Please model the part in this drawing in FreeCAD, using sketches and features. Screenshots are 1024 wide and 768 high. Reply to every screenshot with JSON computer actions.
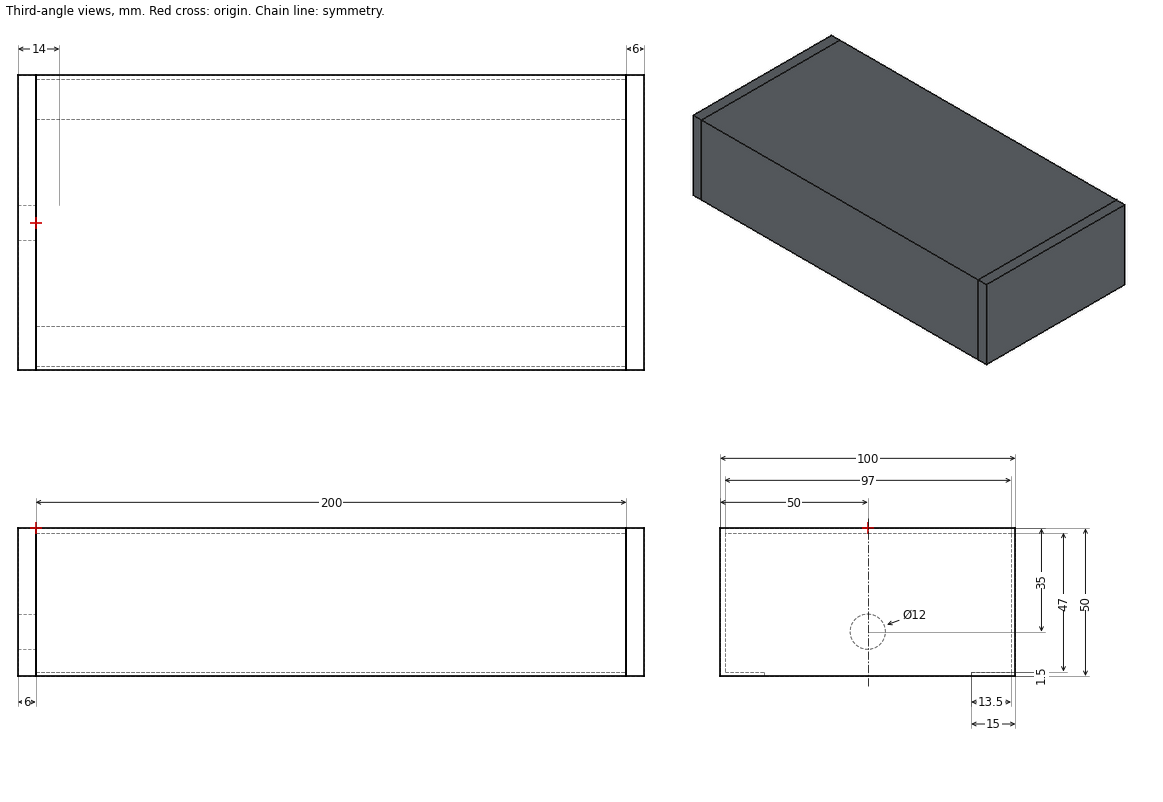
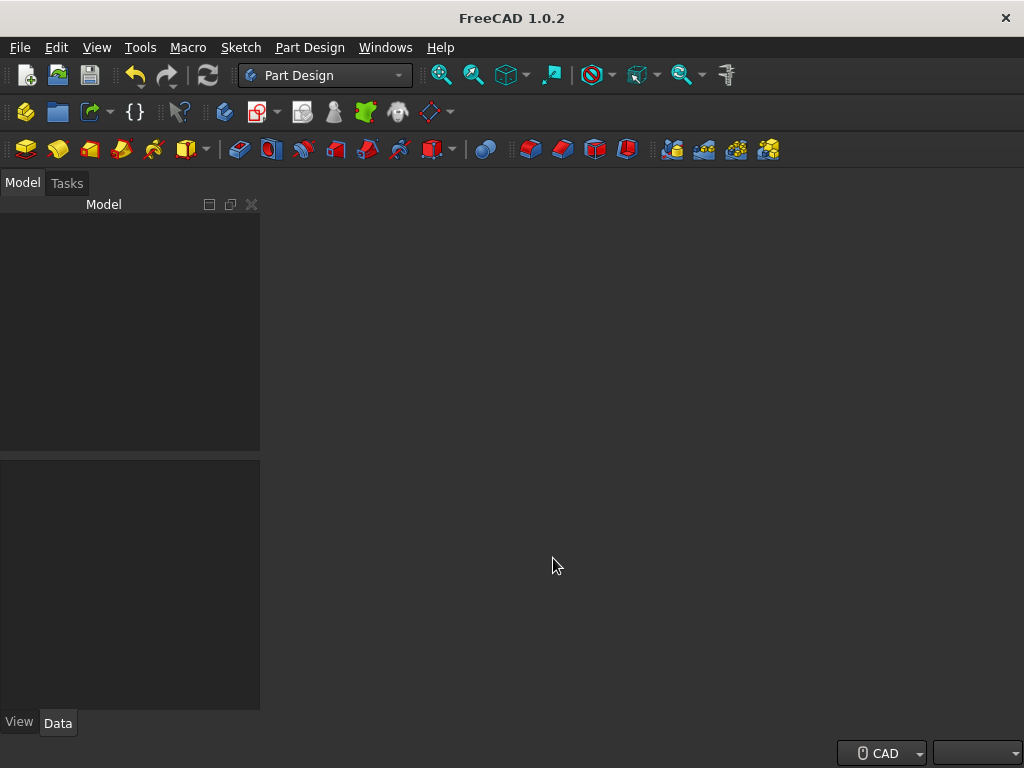
{"action": "left_click", "coordinate": [26, 76]}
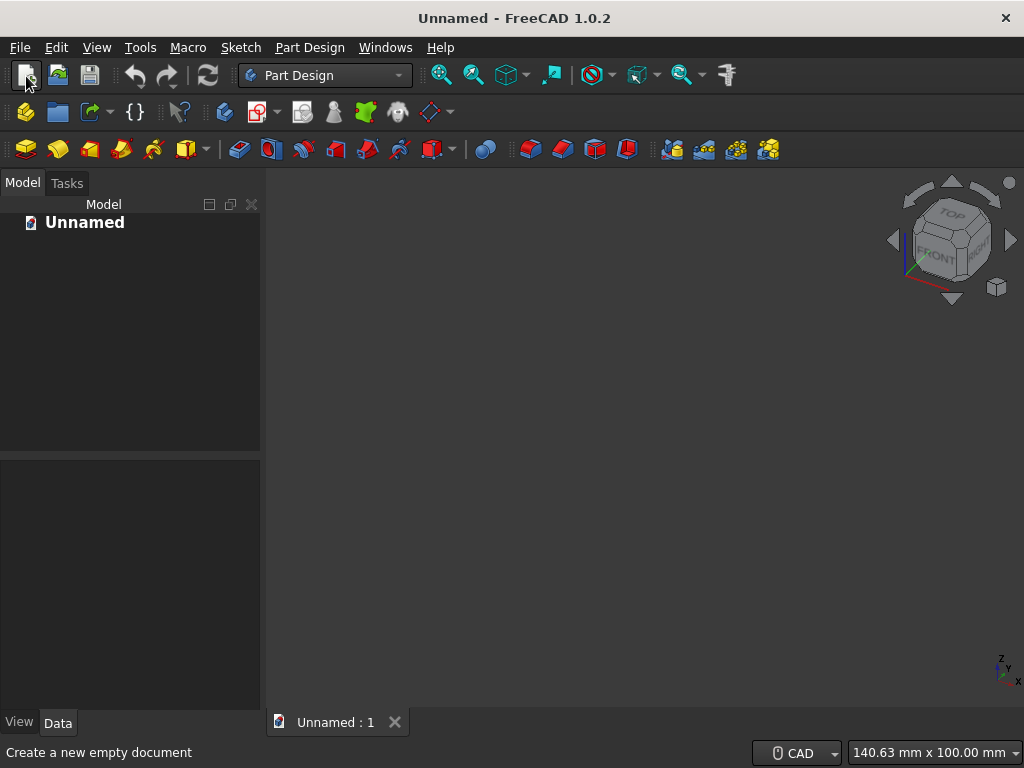
{"action": "left_click", "coordinate": [258, 112]}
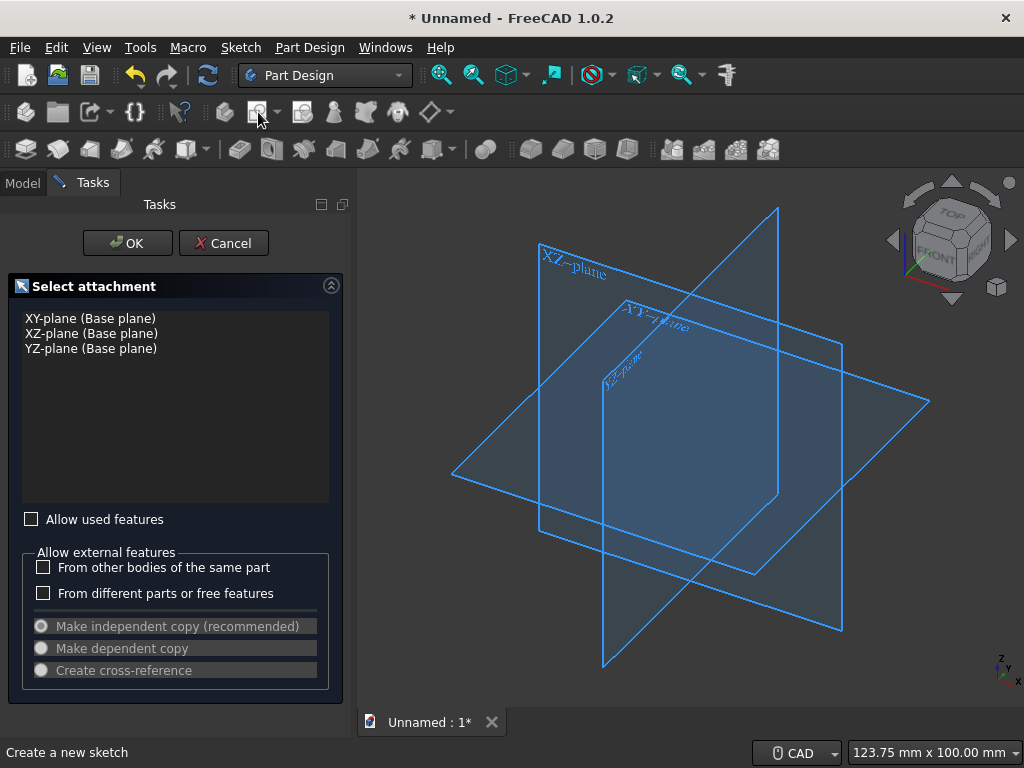
{"action": "left_click", "coordinate": [82, 348]}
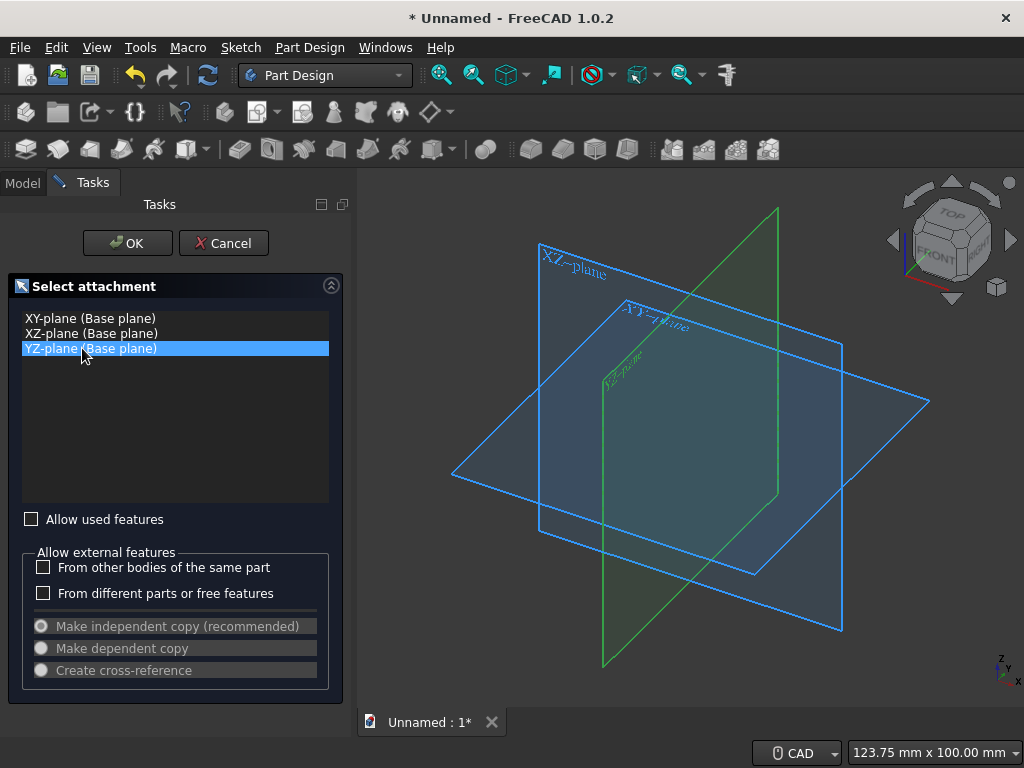
{"action": "left_click", "coordinate": [128, 243]}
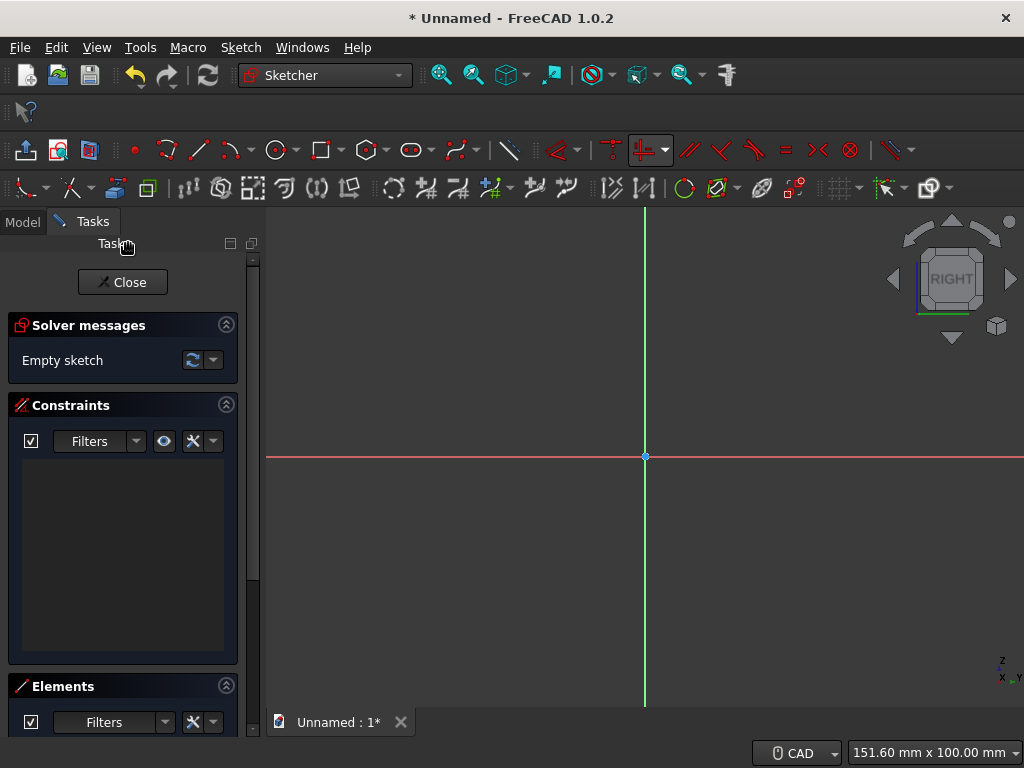
{"action": "scroll", "coordinate": [294, 235], "scroll_direction": "down", "scroll_amount": 1}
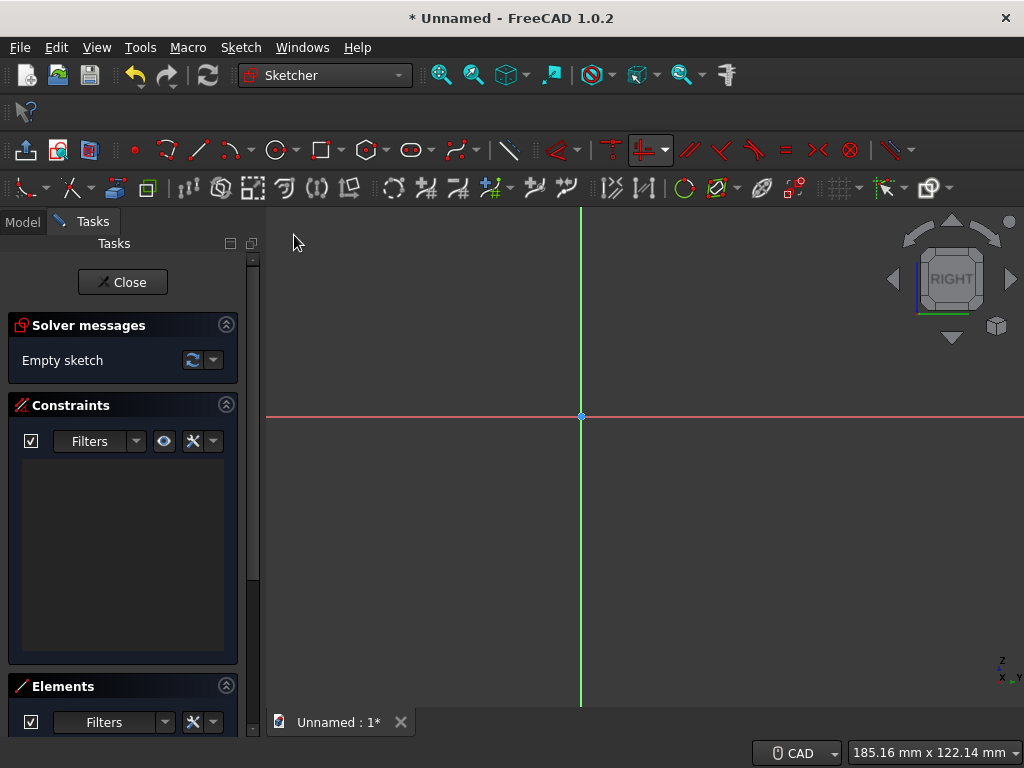
{"action": "left_click", "coordinate": [168, 150]}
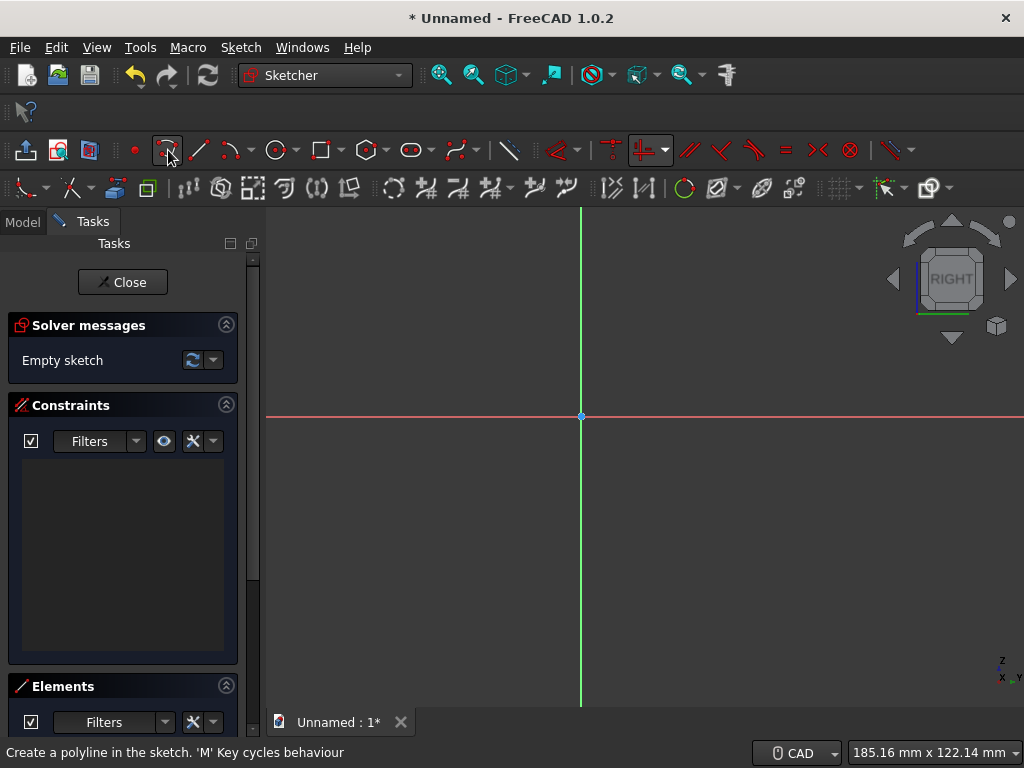
{"action": "scroll", "coordinate": [383, 423], "scroll_direction": "up", "scroll_amount": 5}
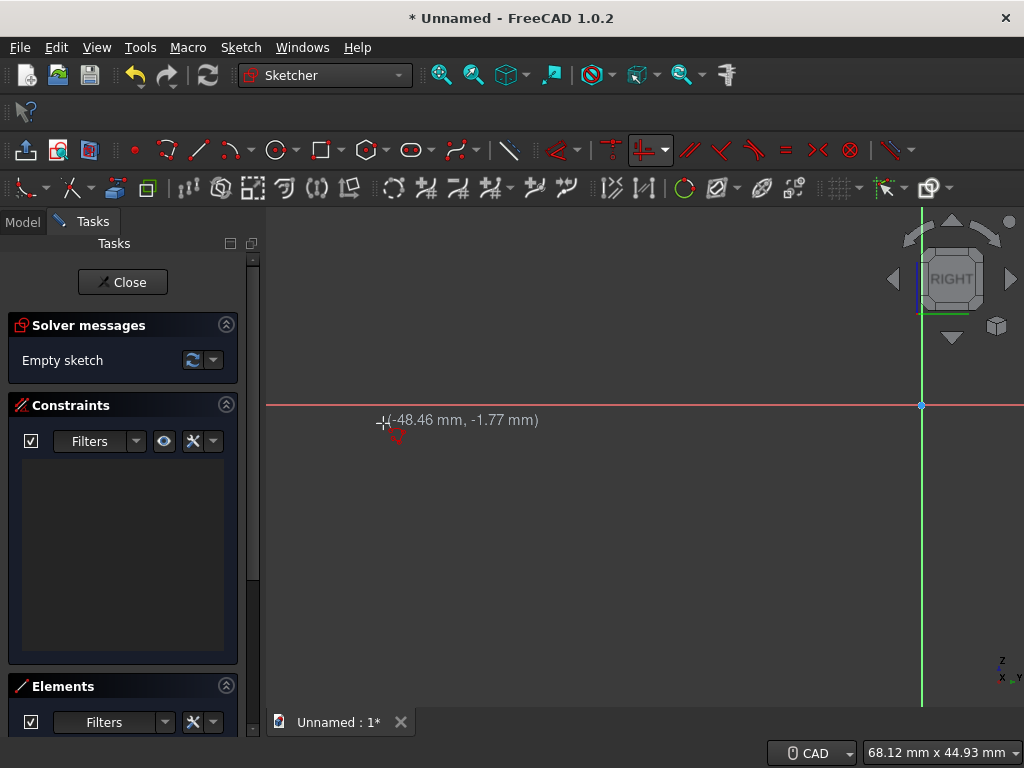
{"action": "left_click", "coordinate": [382, 422]}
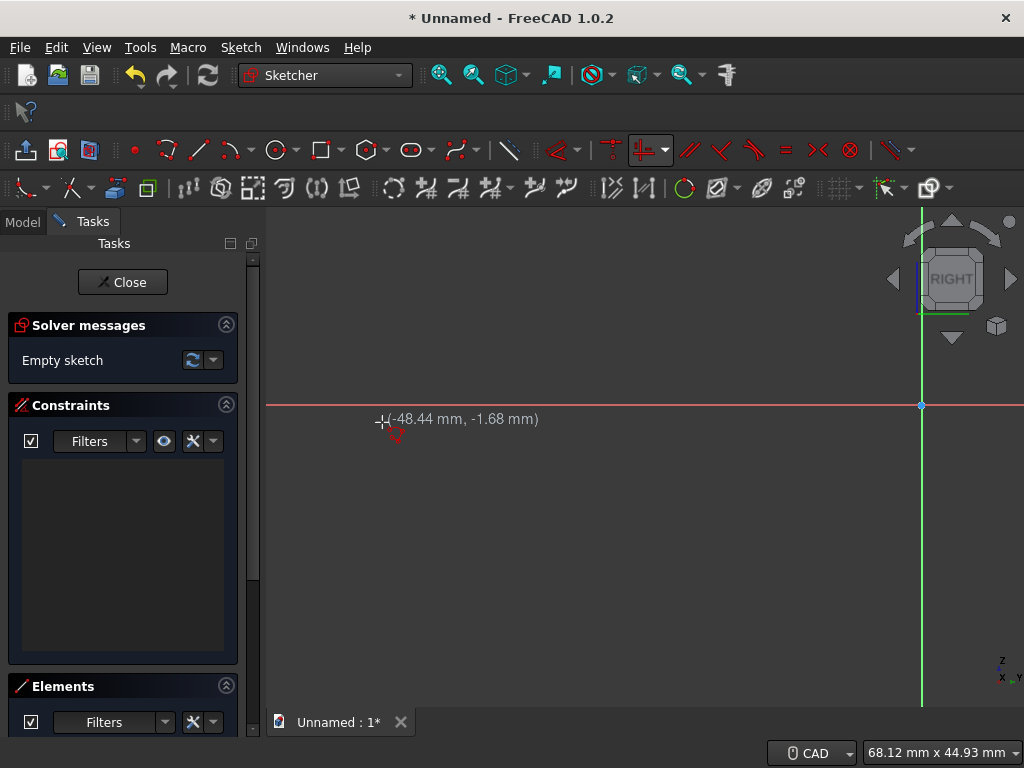
{"action": "scroll", "coordinate": [375, 325], "scroll_direction": "down", "scroll_amount": 5}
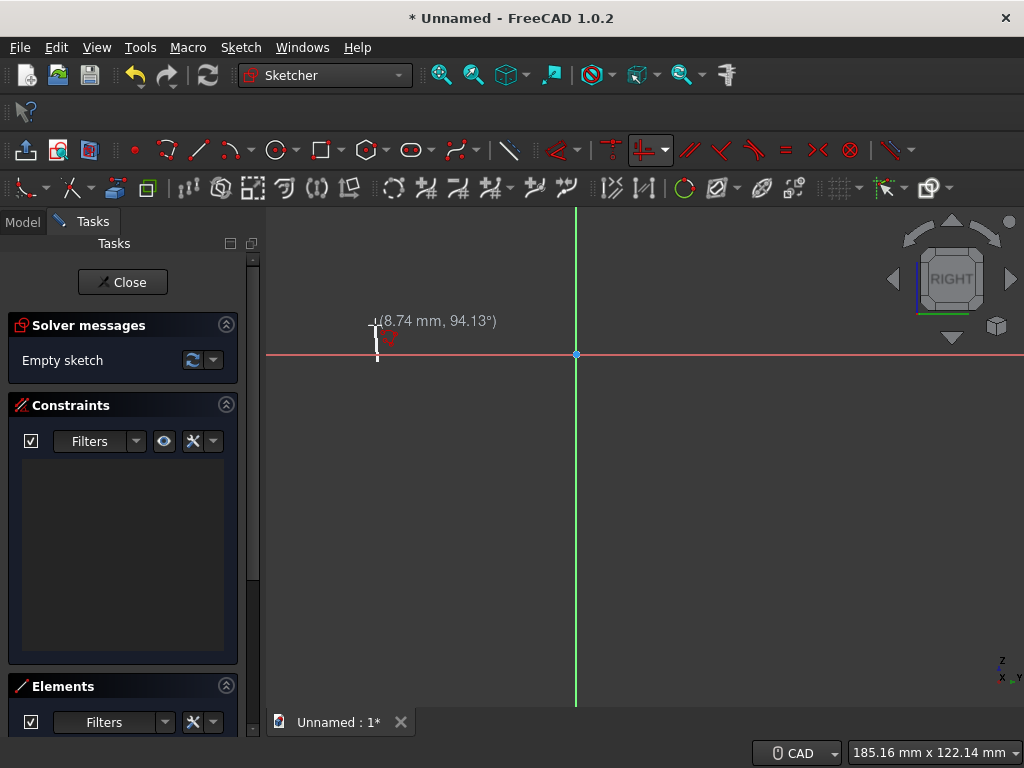
{"action": "scroll", "coordinate": [775, 361], "scroll_direction": "up", "scroll_amount": 5}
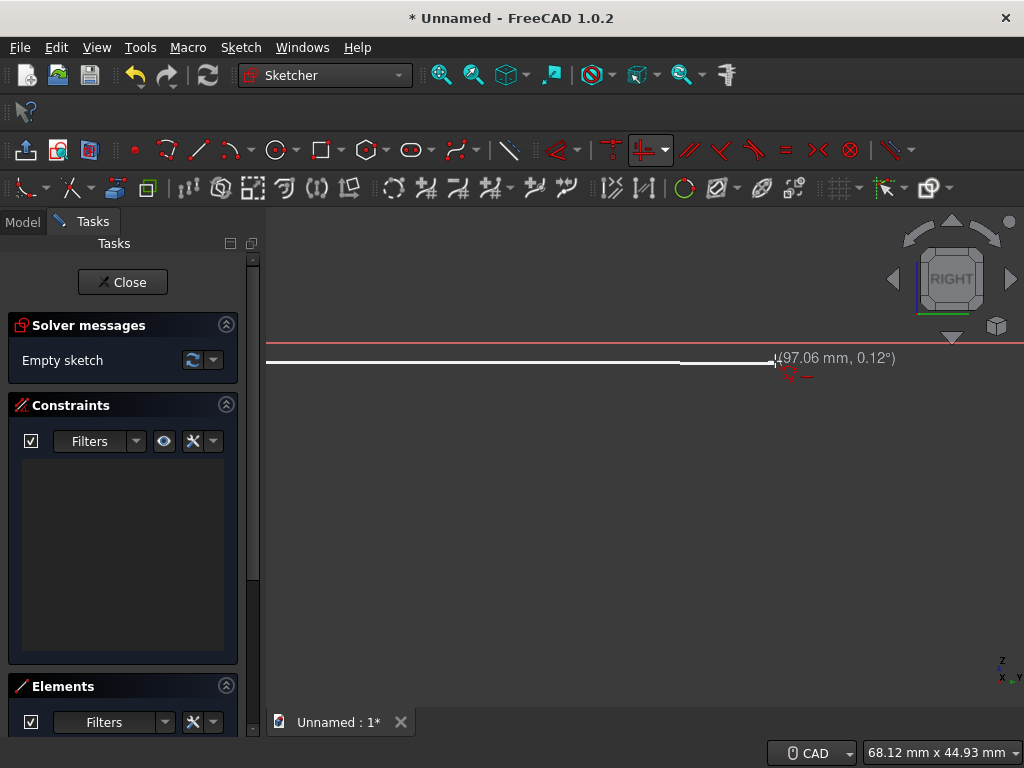
{"action": "left_click", "coordinate": [773, 360]}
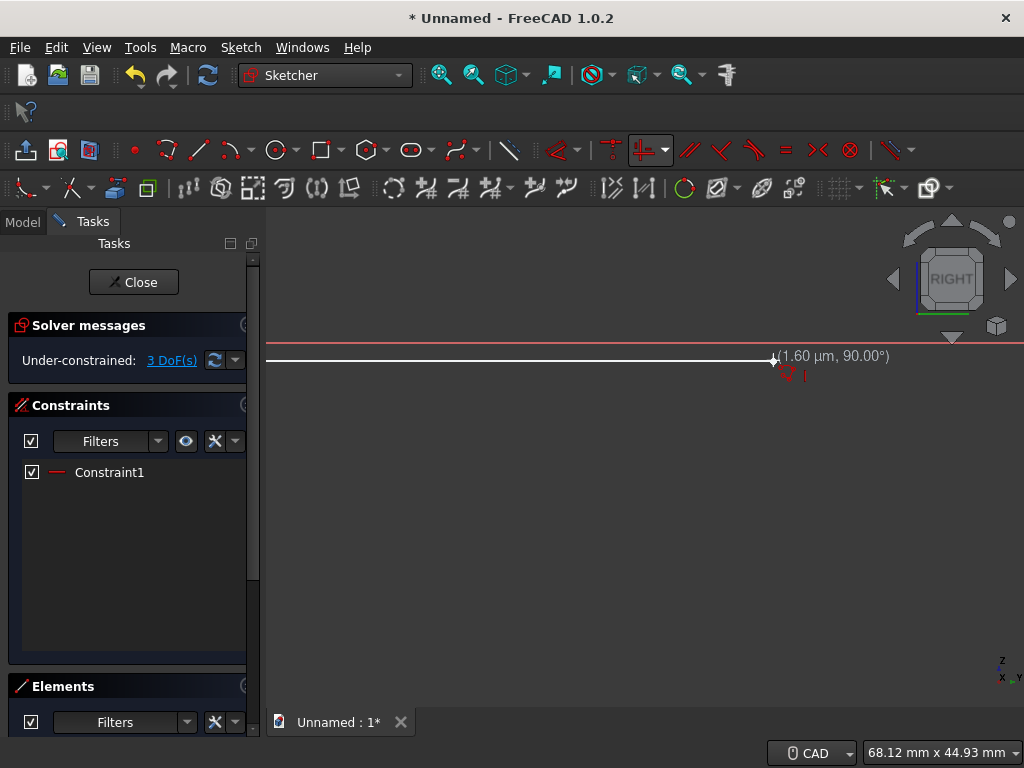
{"action": "scroll", "coordinate": [776, 361], "scroll_direction": "down", "scroll_amount": 5}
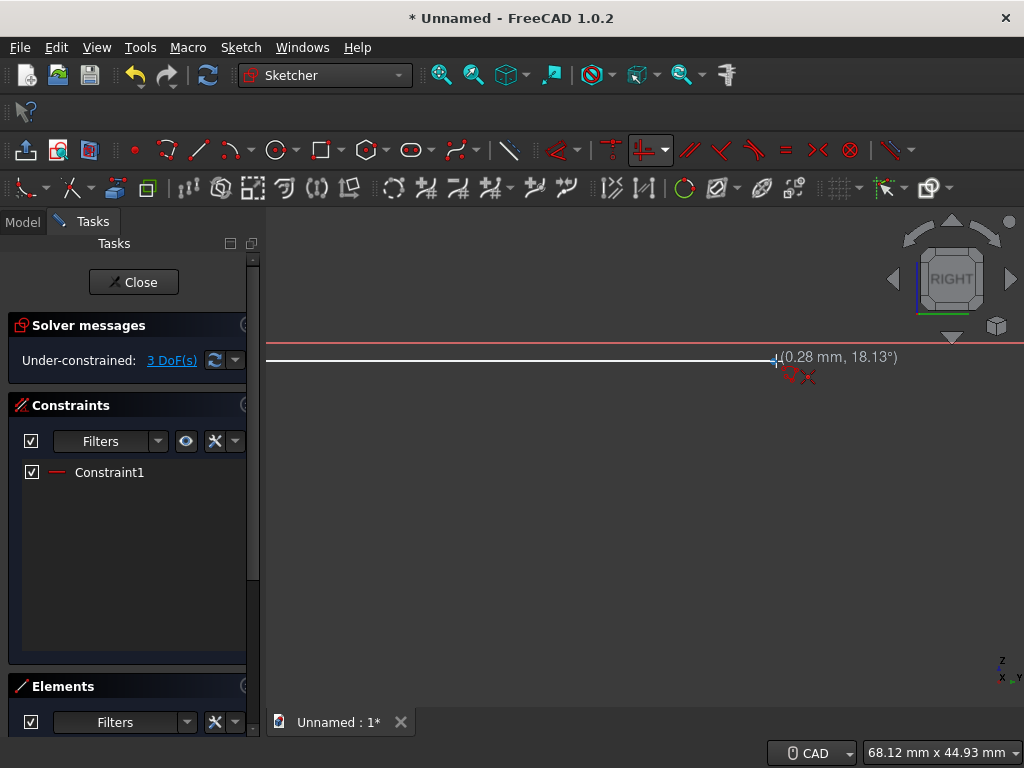
{"action": "left_click", "coordinate": [775, 553]}
{"action": "left_click", "coordinate": [720, 553]}